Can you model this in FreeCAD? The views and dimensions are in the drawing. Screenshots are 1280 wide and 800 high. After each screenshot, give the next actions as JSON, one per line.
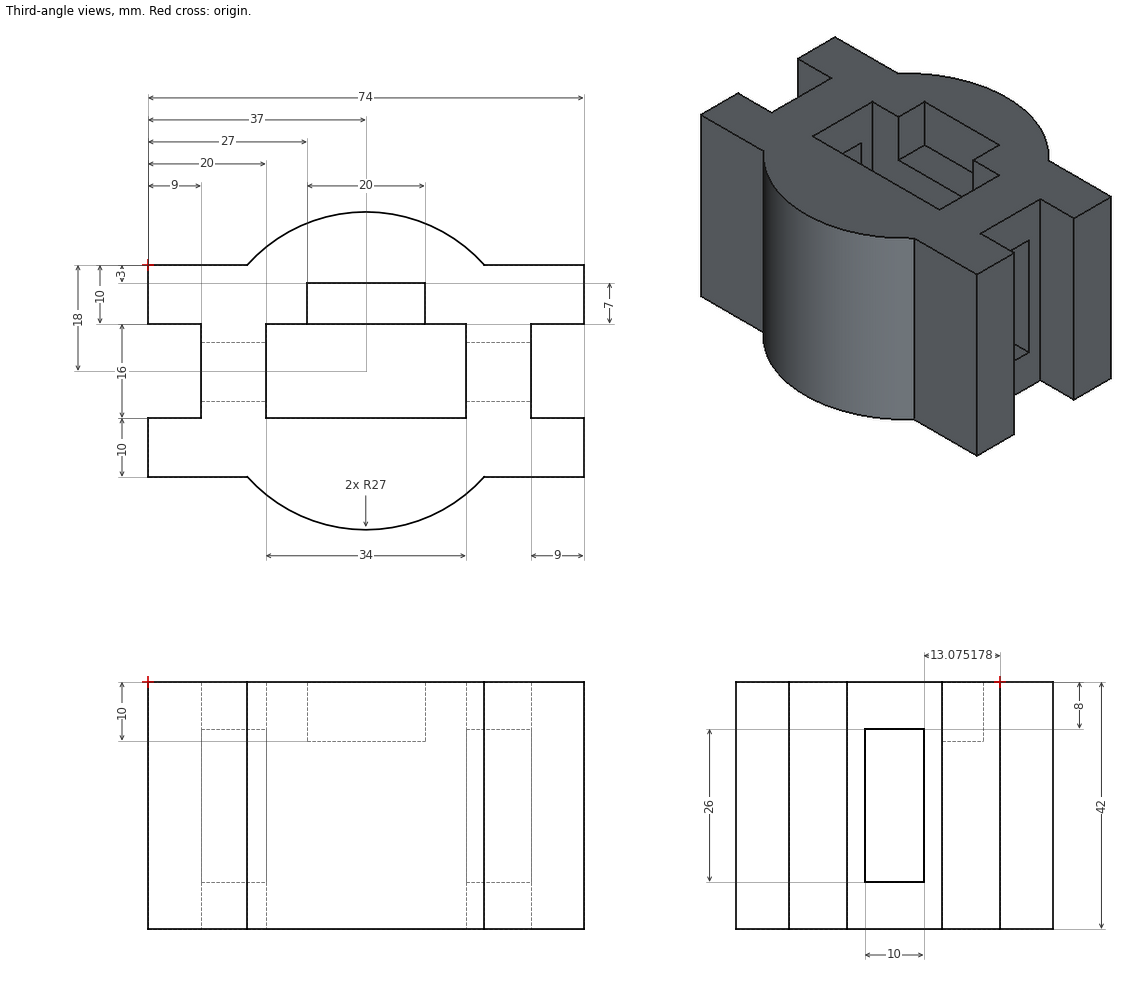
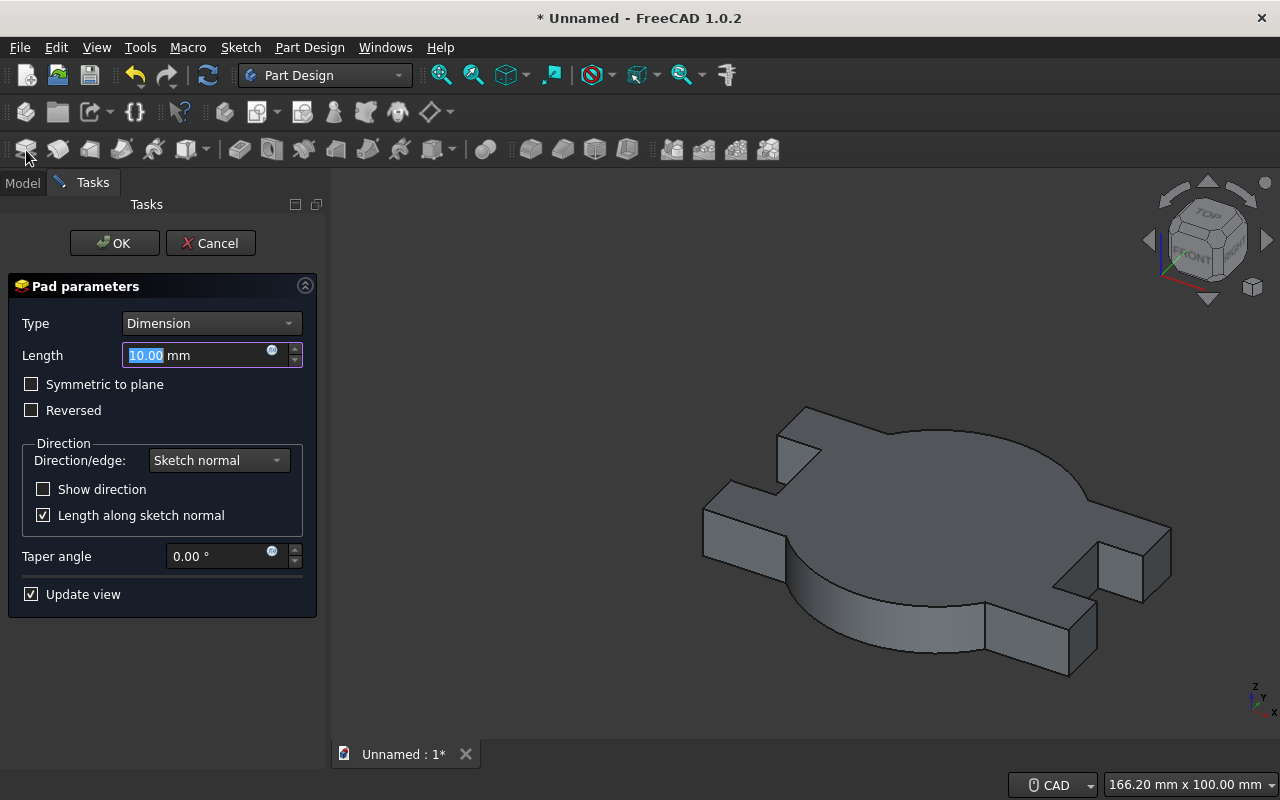
{"action": "type", "text": "42"}
{"action": "key", "text": "Tab"}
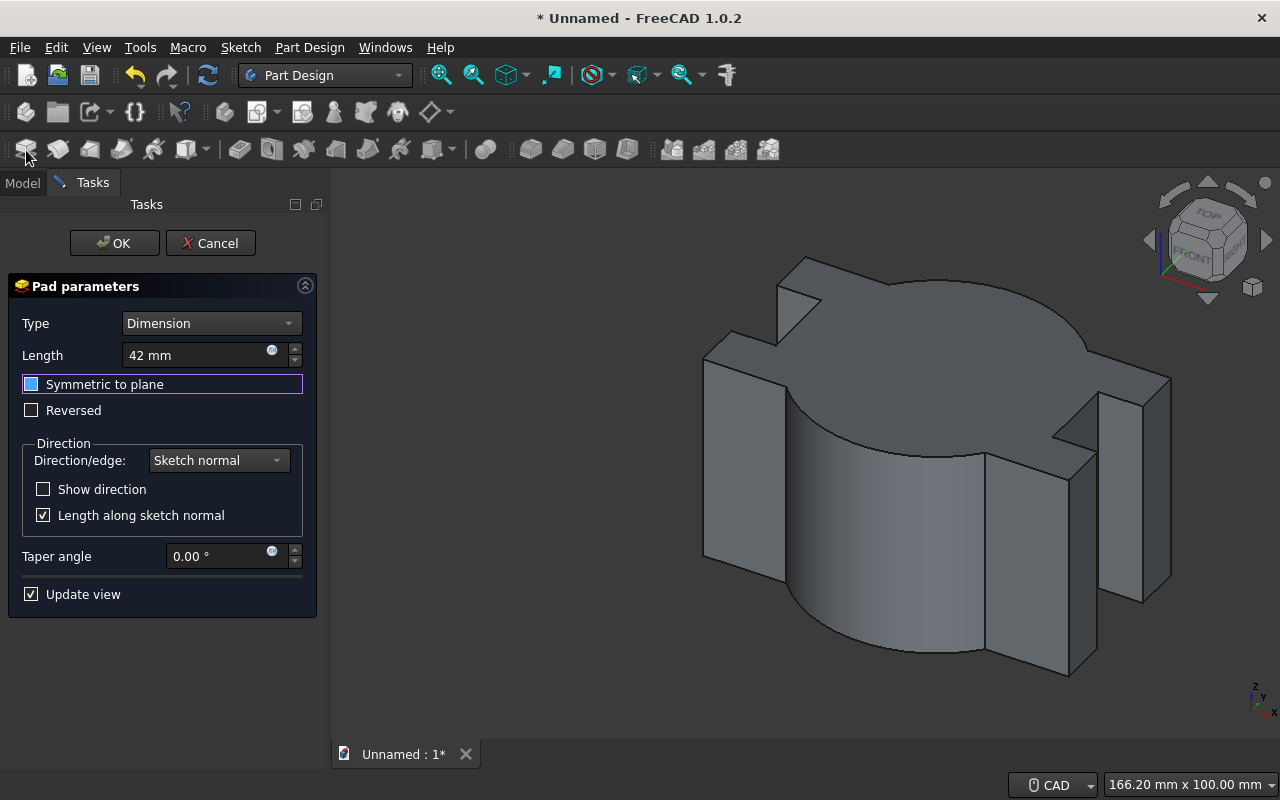
{"action": "left_click", "coordinate": [30, 410]}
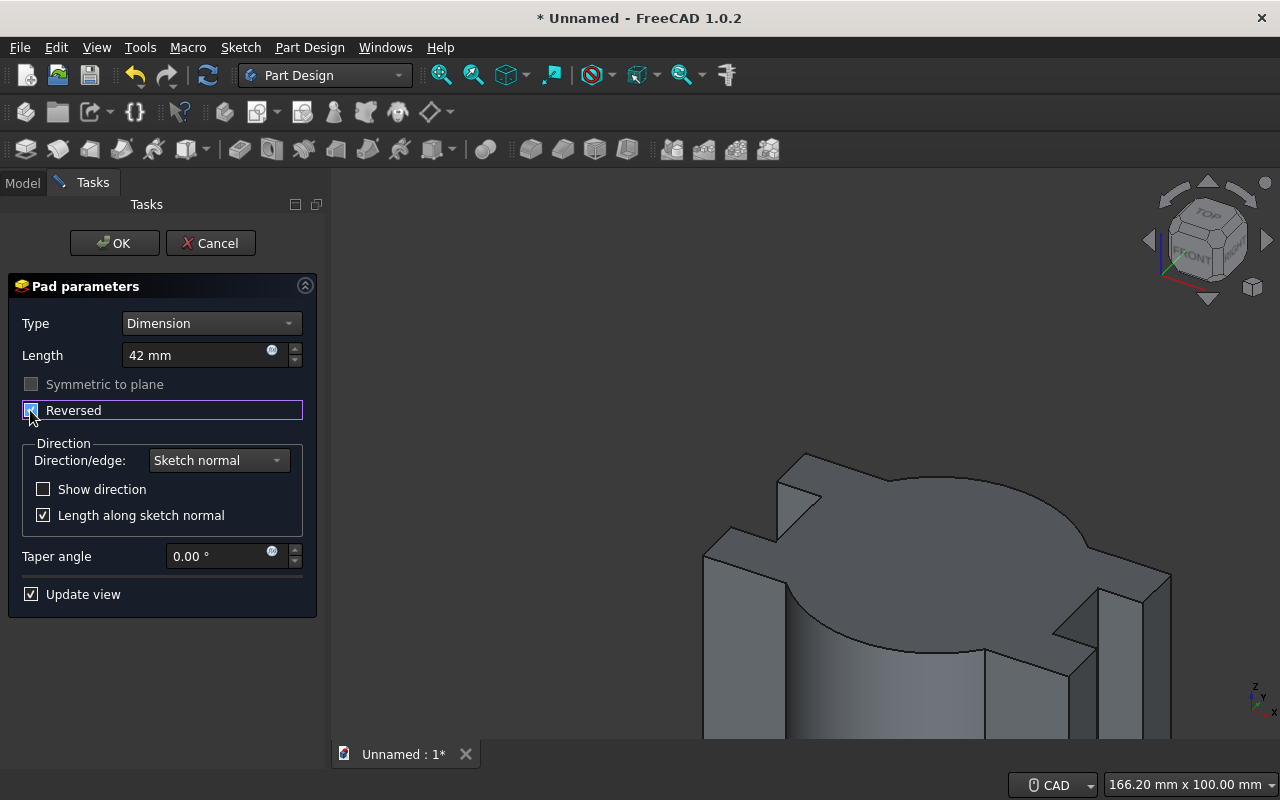
{"action": "left_click", "coordinate": [115, 243]}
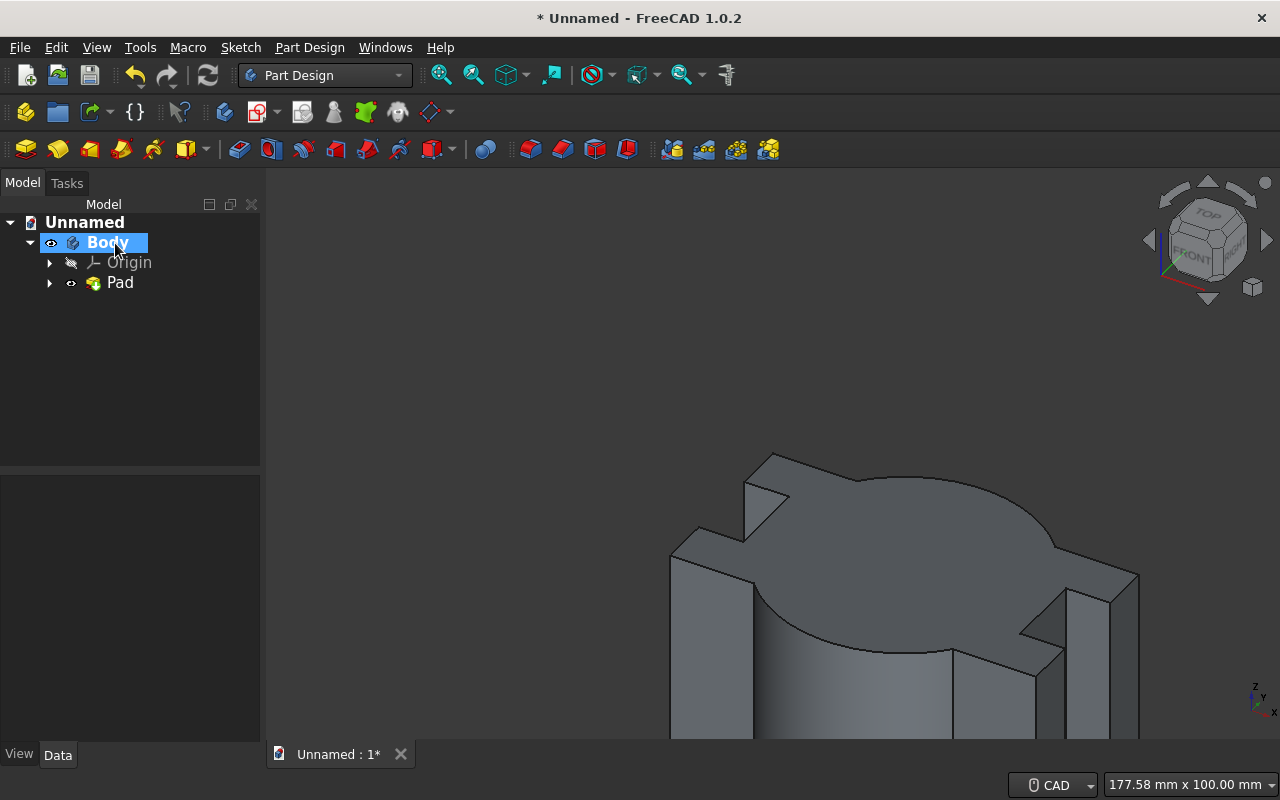
{"action": "left_click", "coordinate": [442, 76]}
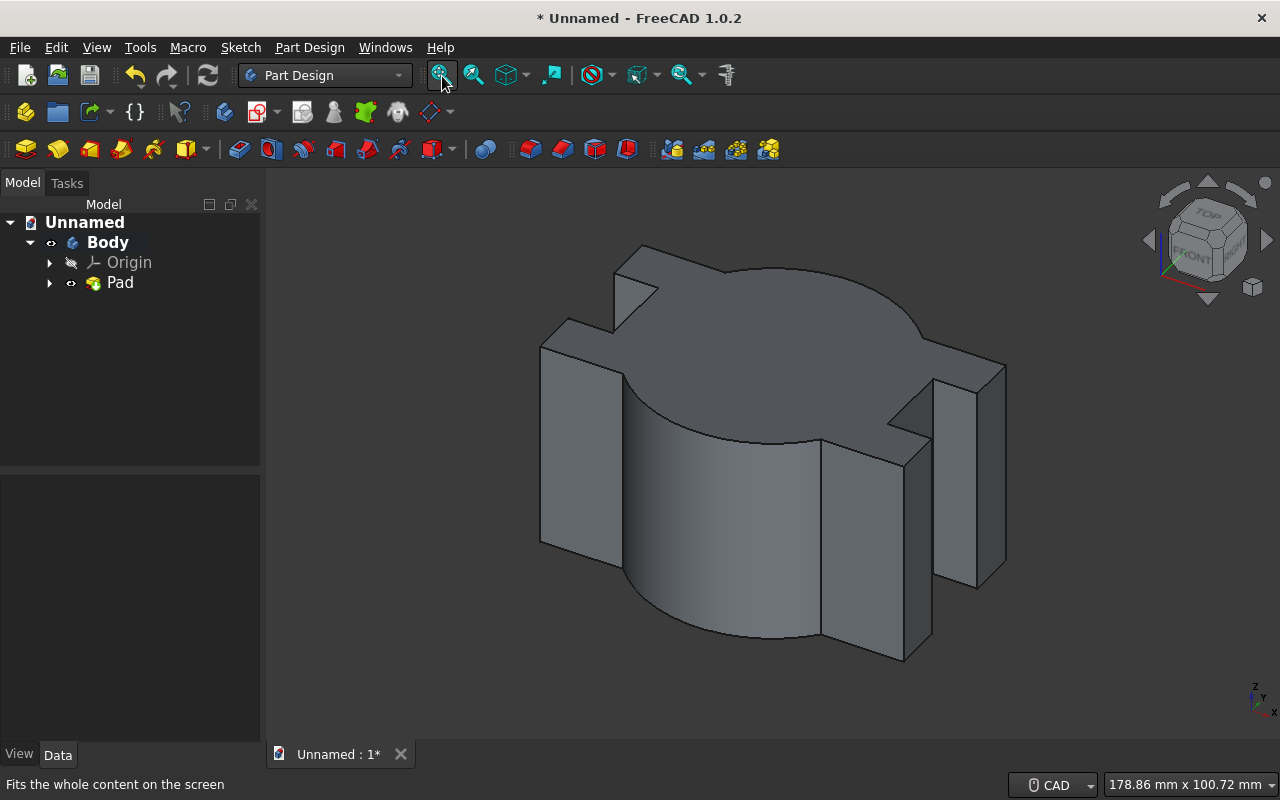
{"action": "left_click", "coordinate": [258, 112]}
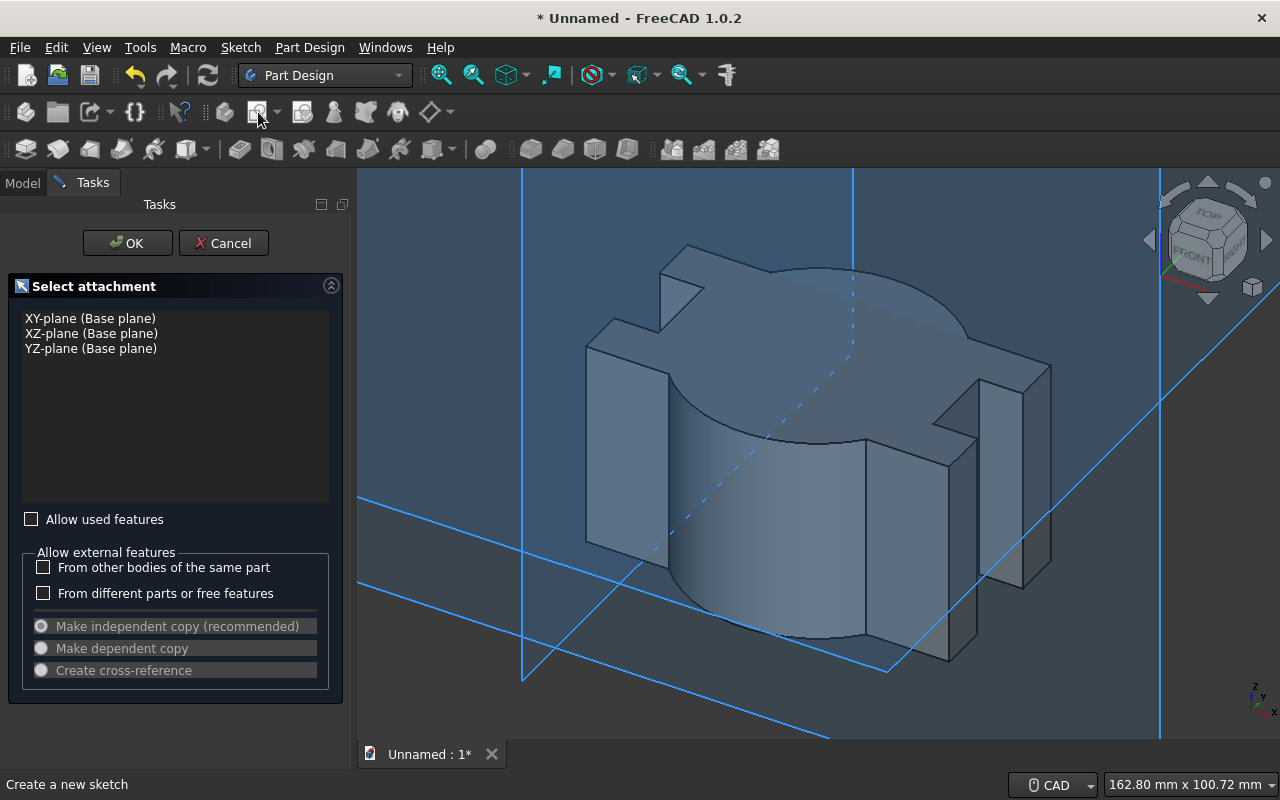
{"action": "left_click", "coordinate": [82, 318]}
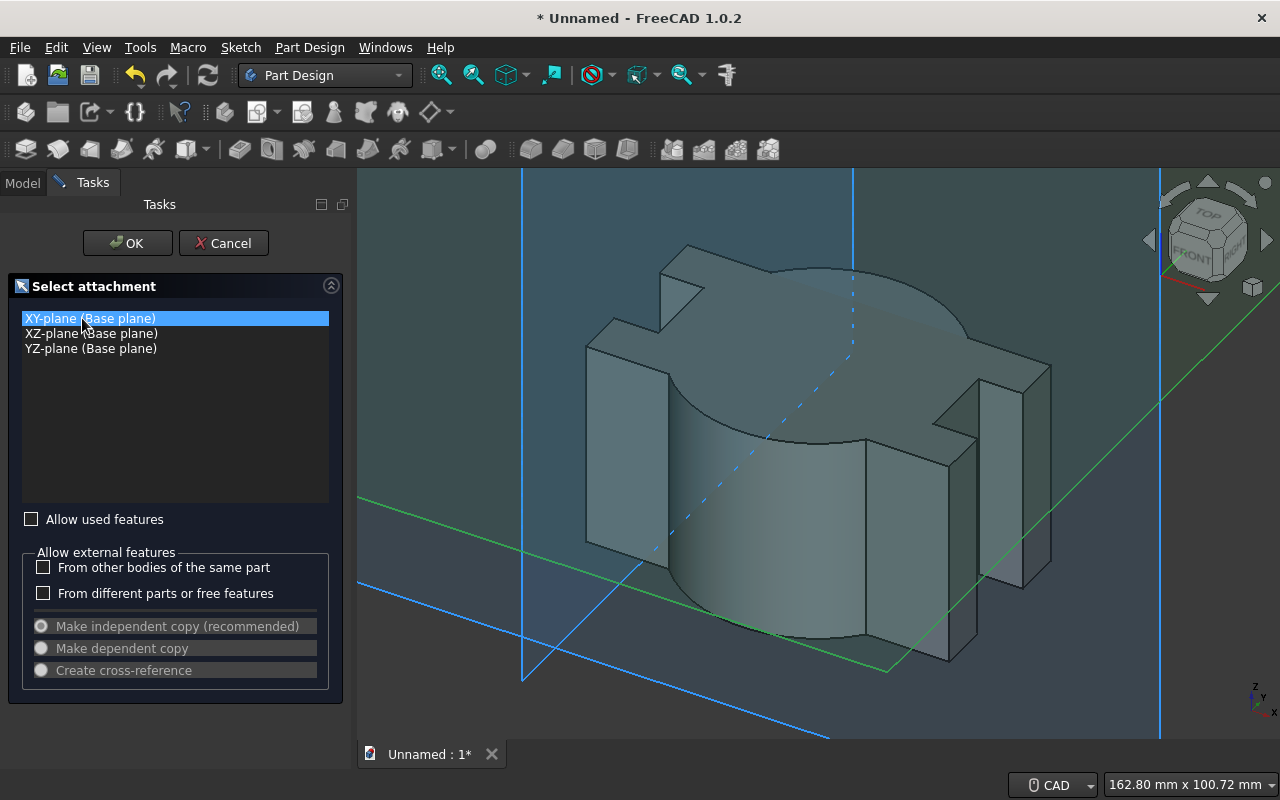
{"action": "left_click", "coordinate": [128, 243]}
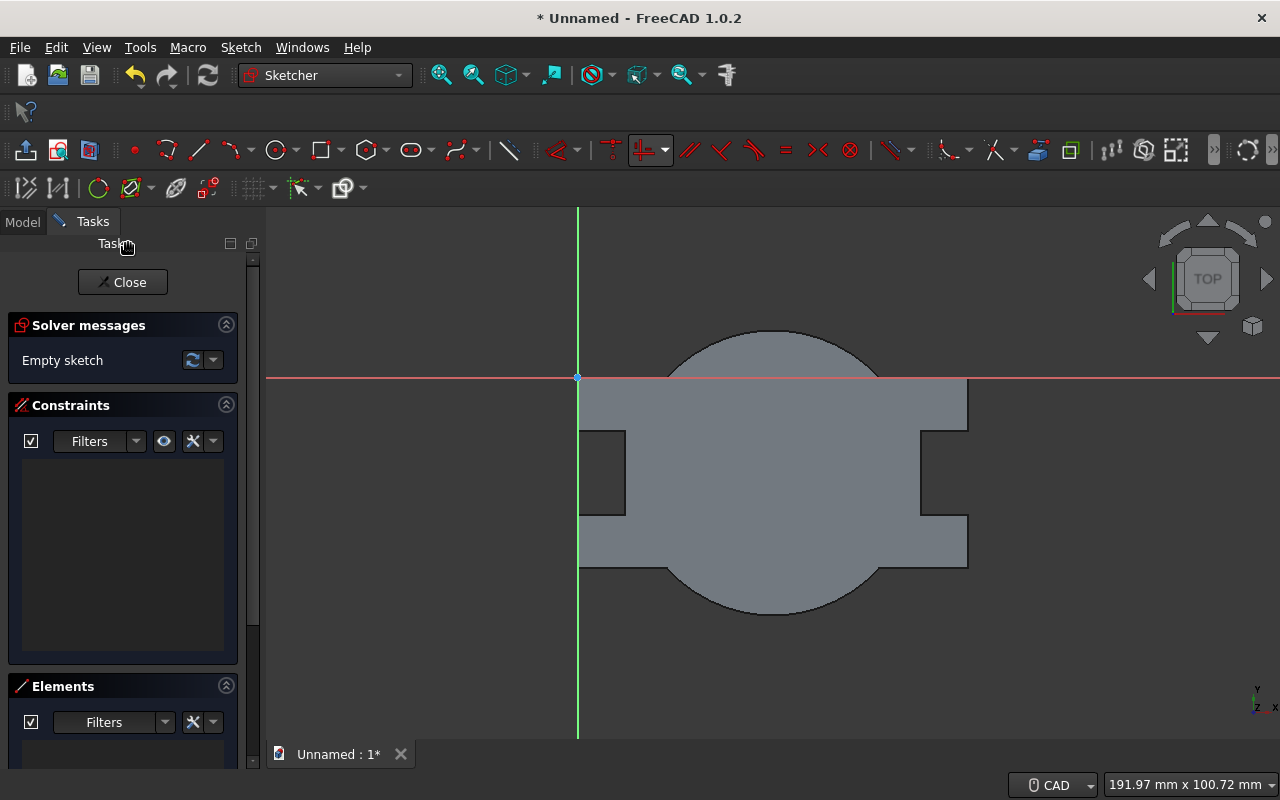
{"action": "scroll", "coordinate": [733, 425], "scroll_direction": "up", "scroll_amount": 4}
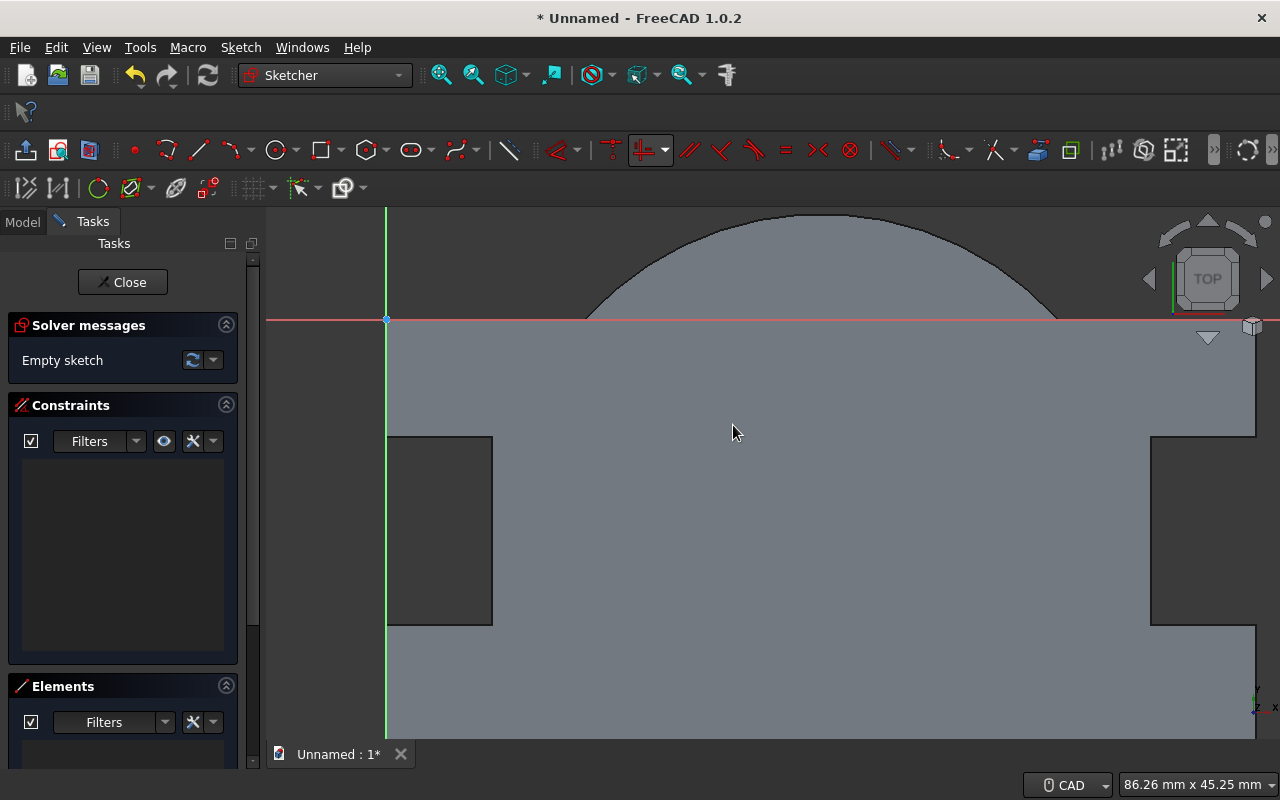
{"action": "left_click", "coordinate": [322, 150]}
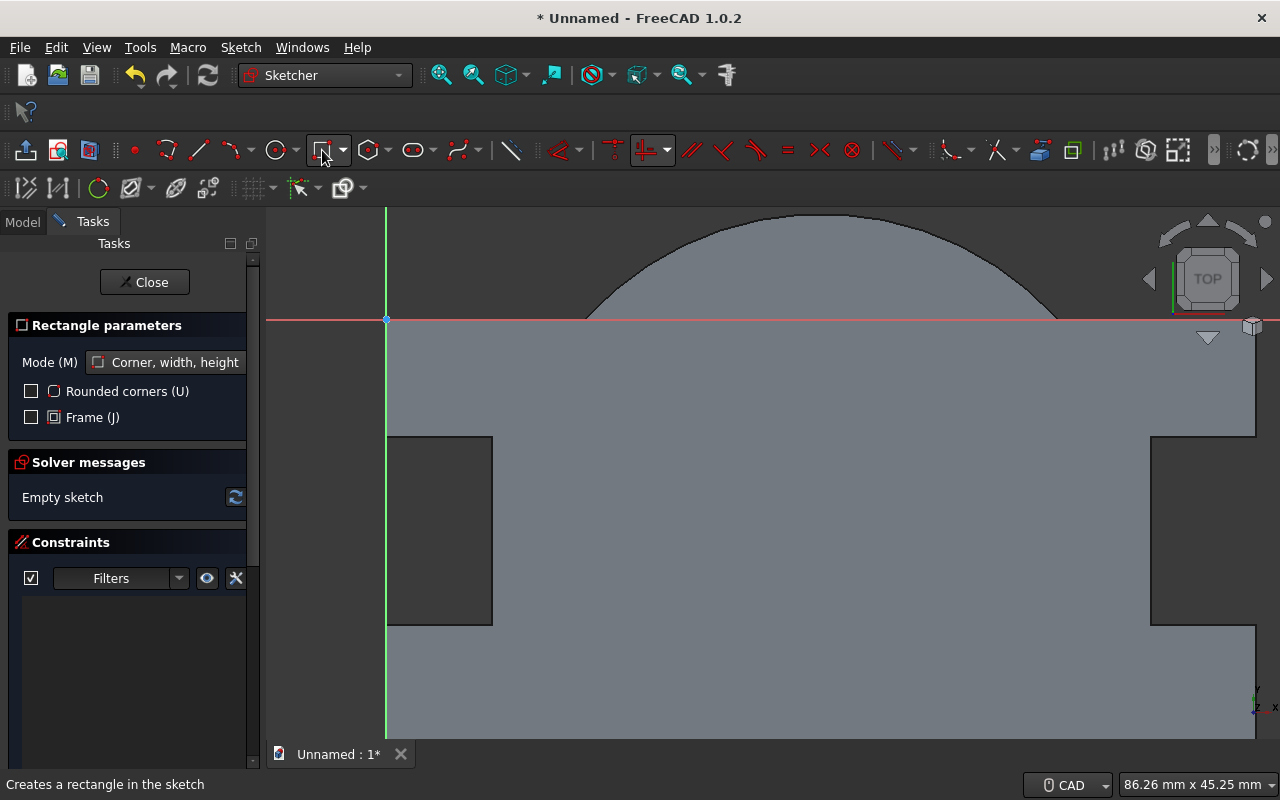
{"action": "left_click", "coordinate": [622, 437]}
{"action": "mouse_move", "coordinate": [1021, 625]}